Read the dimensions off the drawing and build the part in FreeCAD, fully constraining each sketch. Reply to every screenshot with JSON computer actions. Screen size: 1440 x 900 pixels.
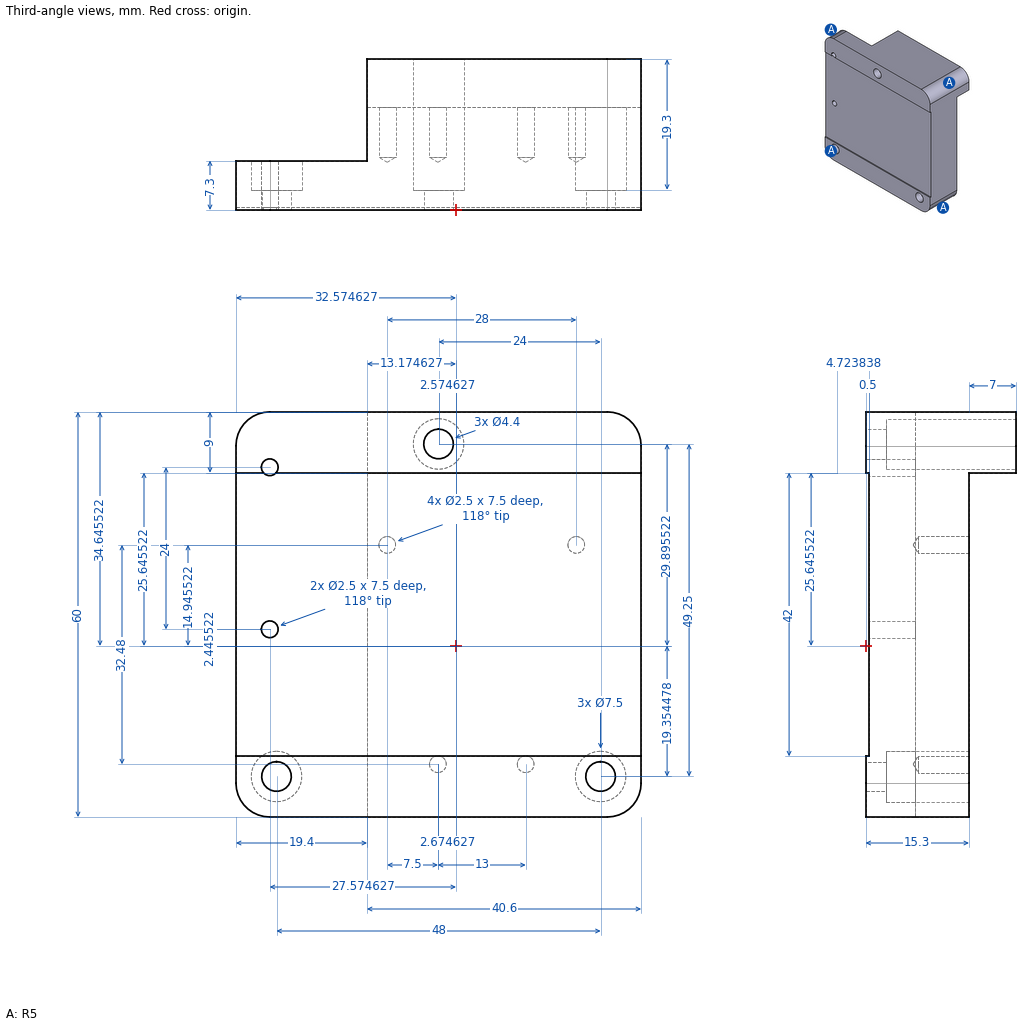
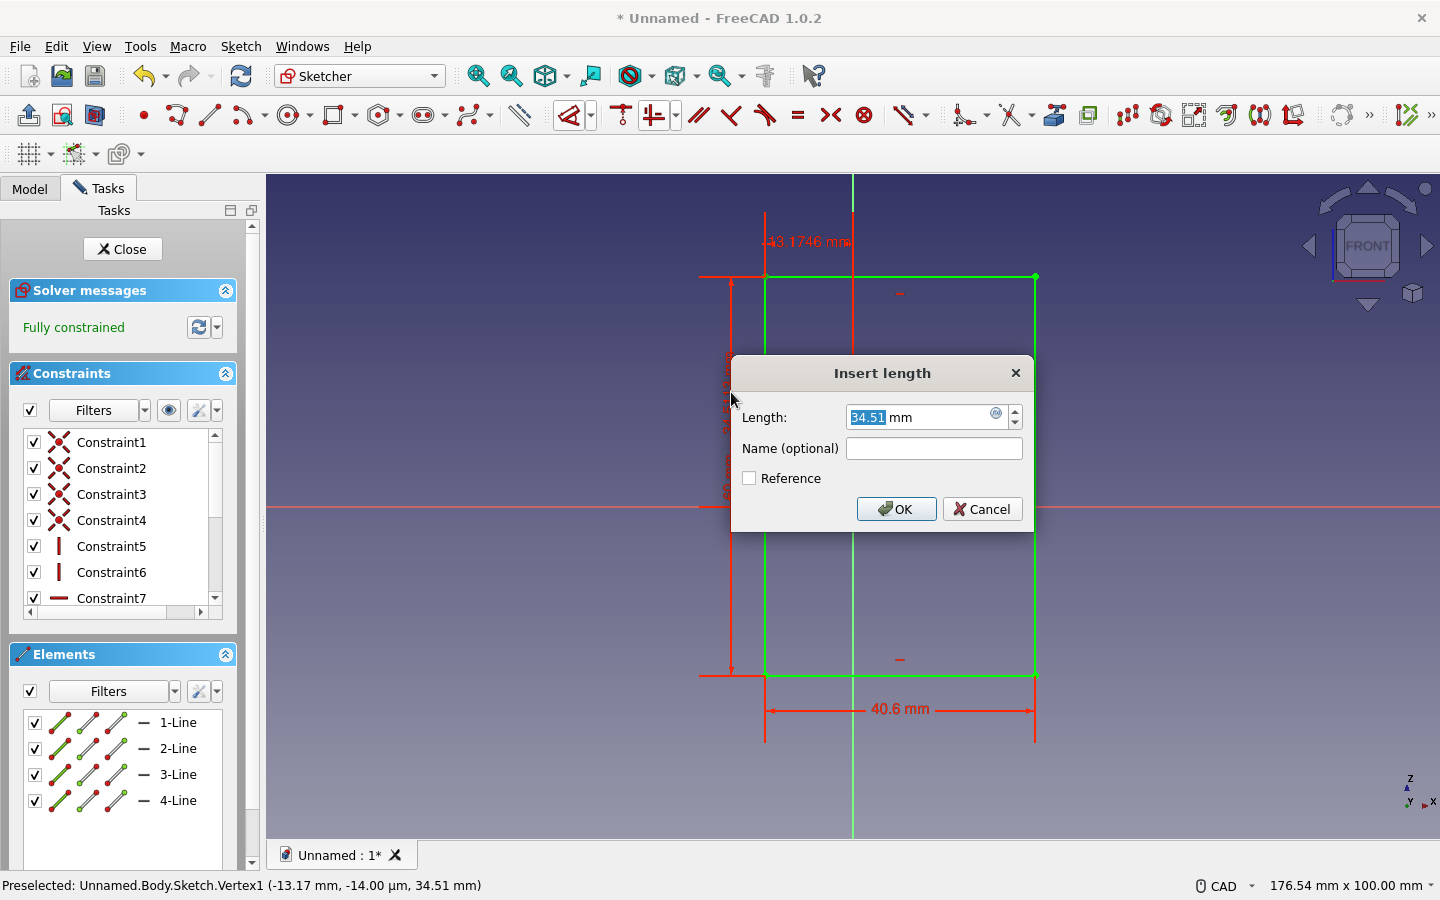
{"action": "type", "text": "34.645522"}
{"action": "key", "text": "Return"}
{"action": "key", "text": "Escape"}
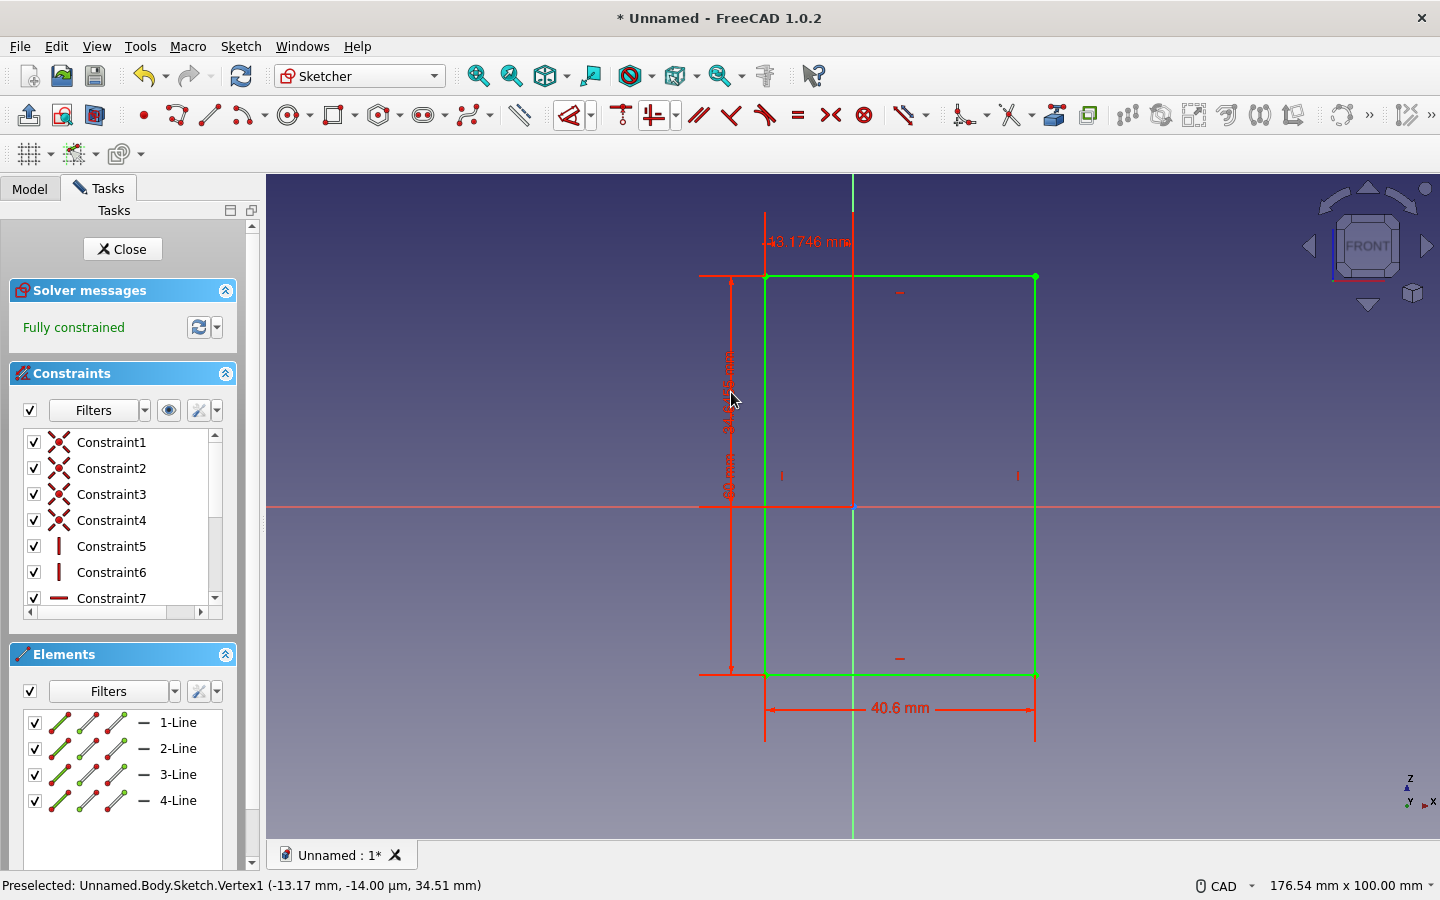
{"action": "left_click", "coordinate": [123, 249]}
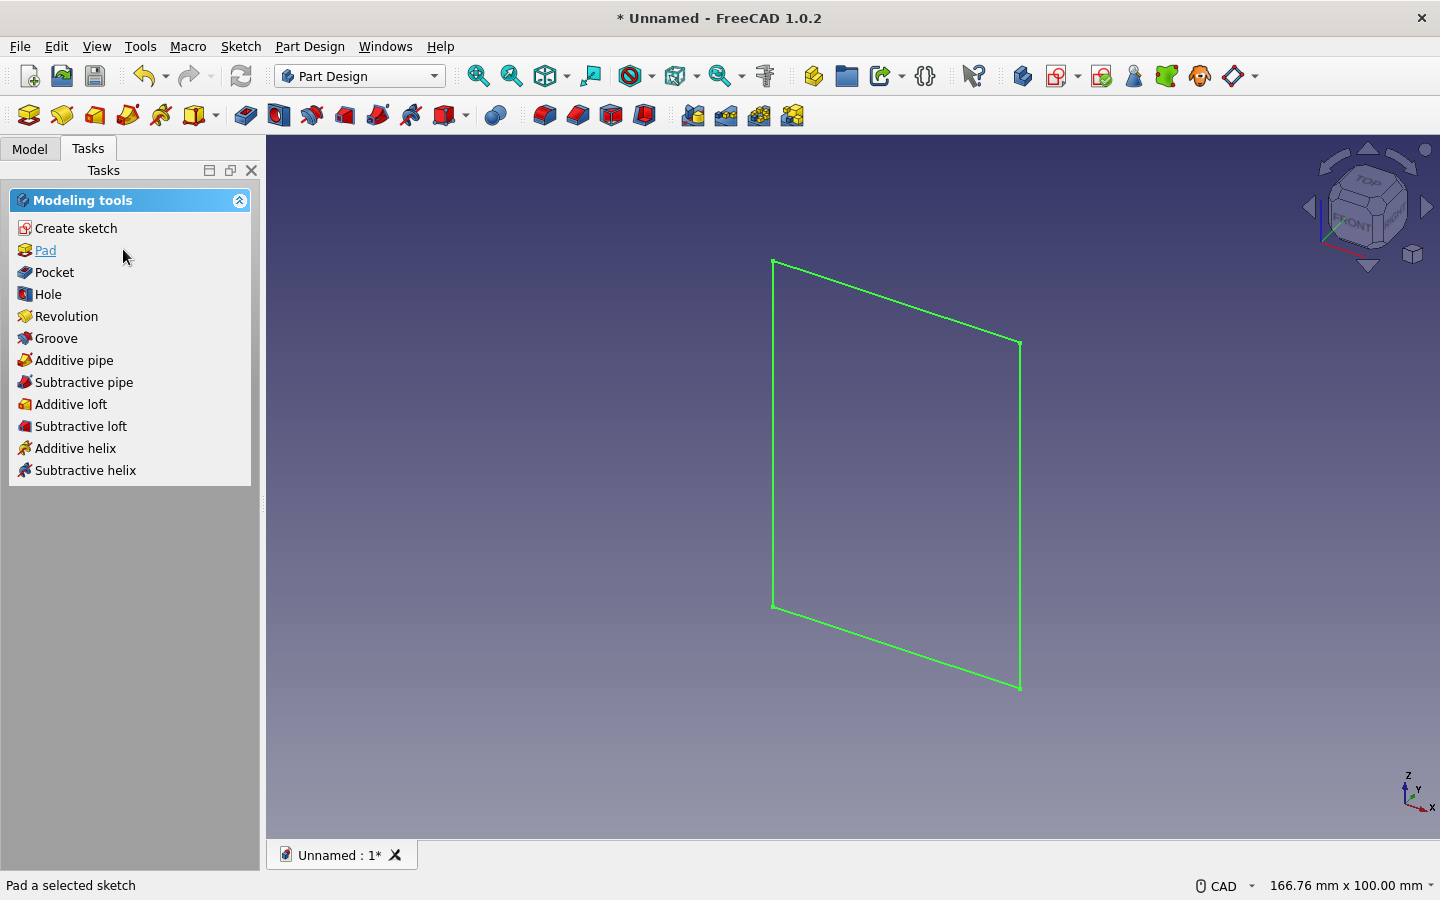
{"action": "left_click", "coordinate": [29, 116]}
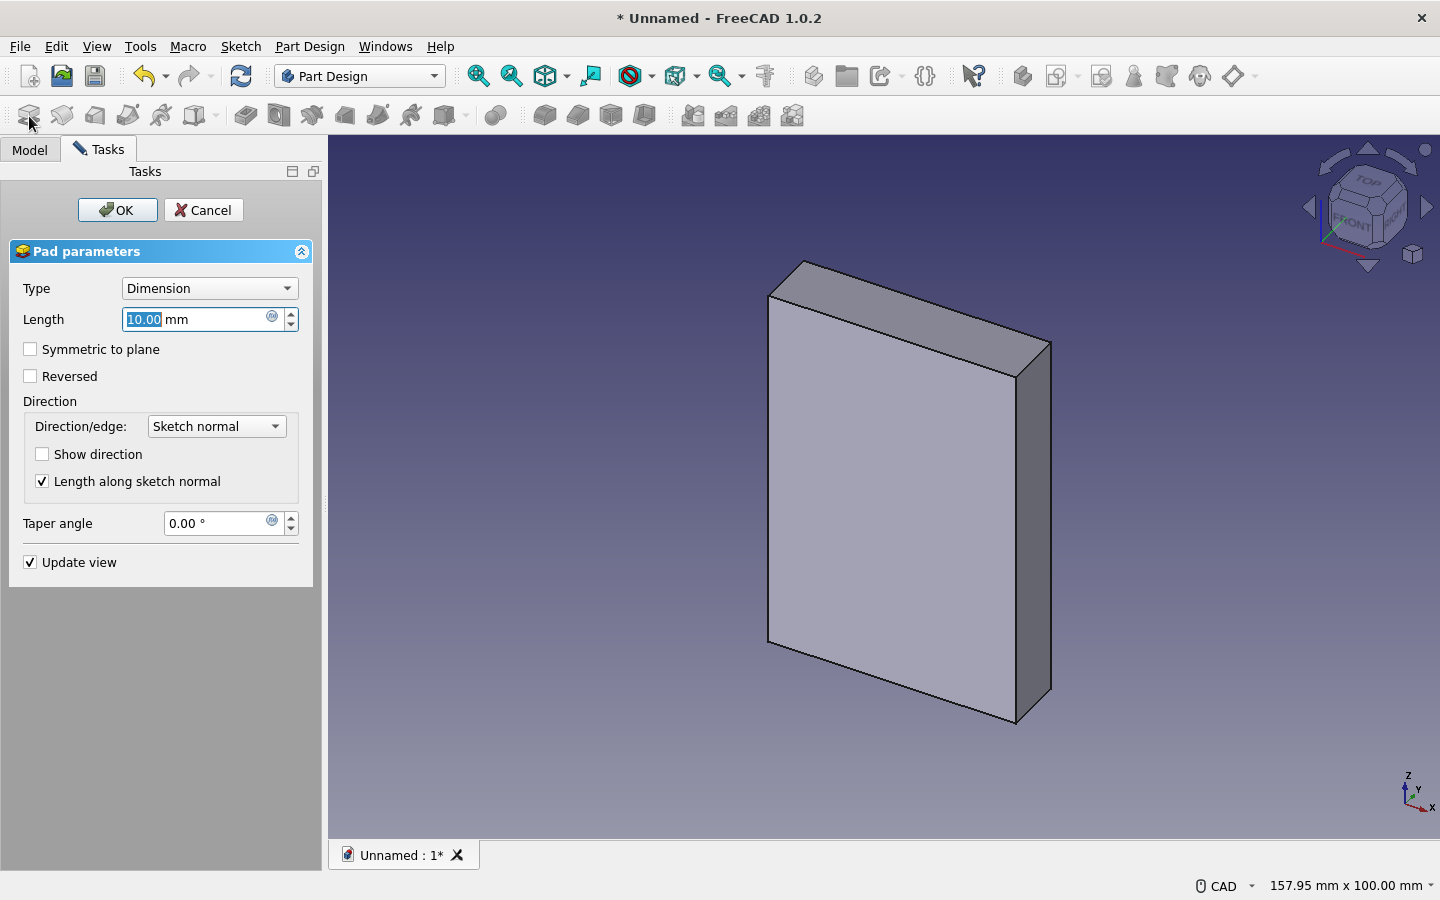
{"action": "type", "text": "15.3"}
{"action": "key", "text": "Tab"}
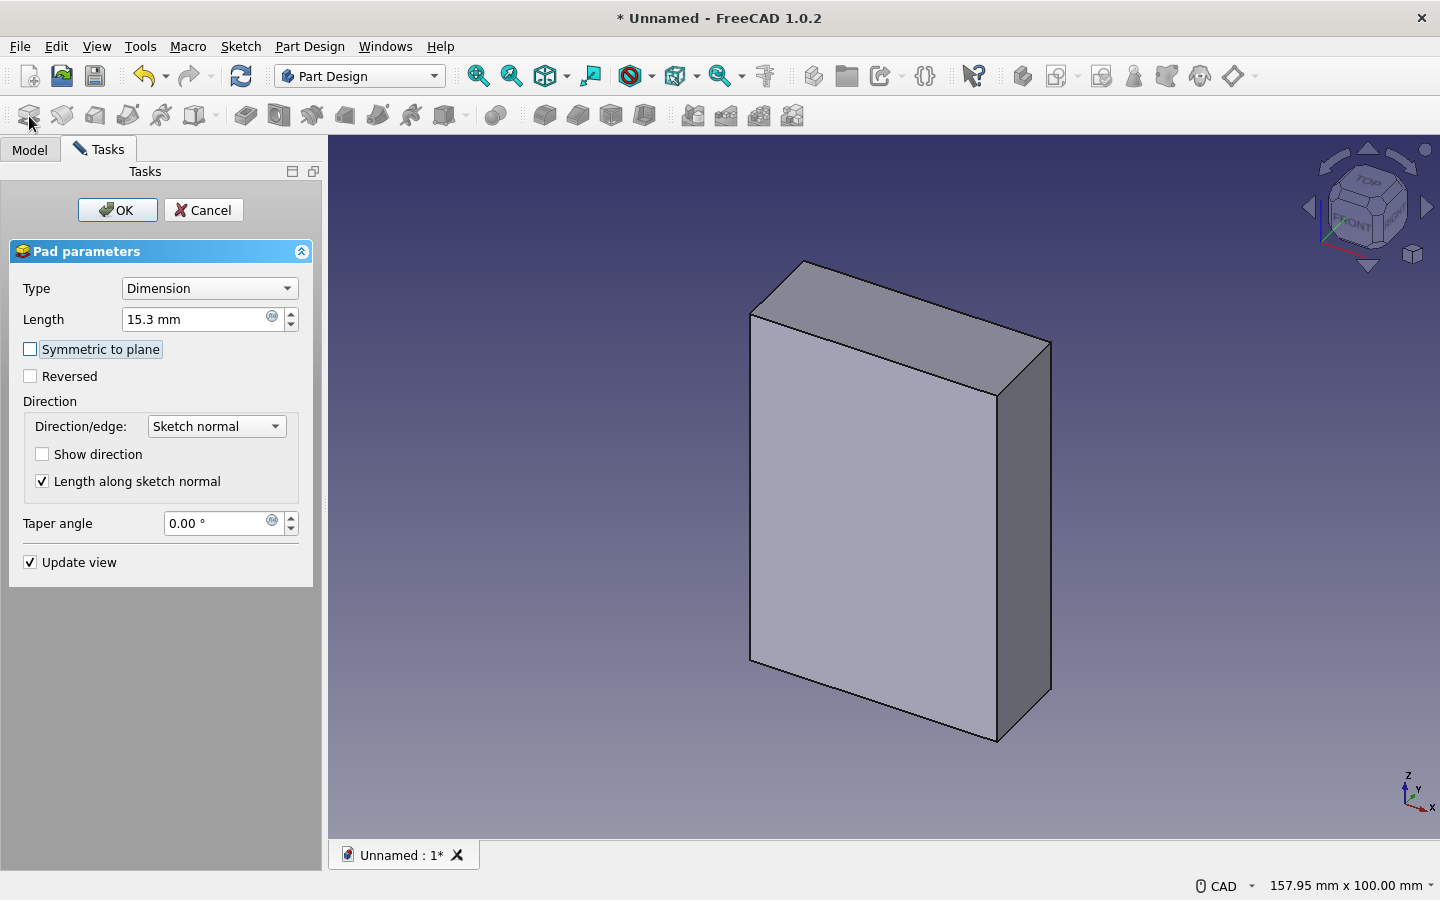
{"action": "left_click", "coordinate": [31, 376]}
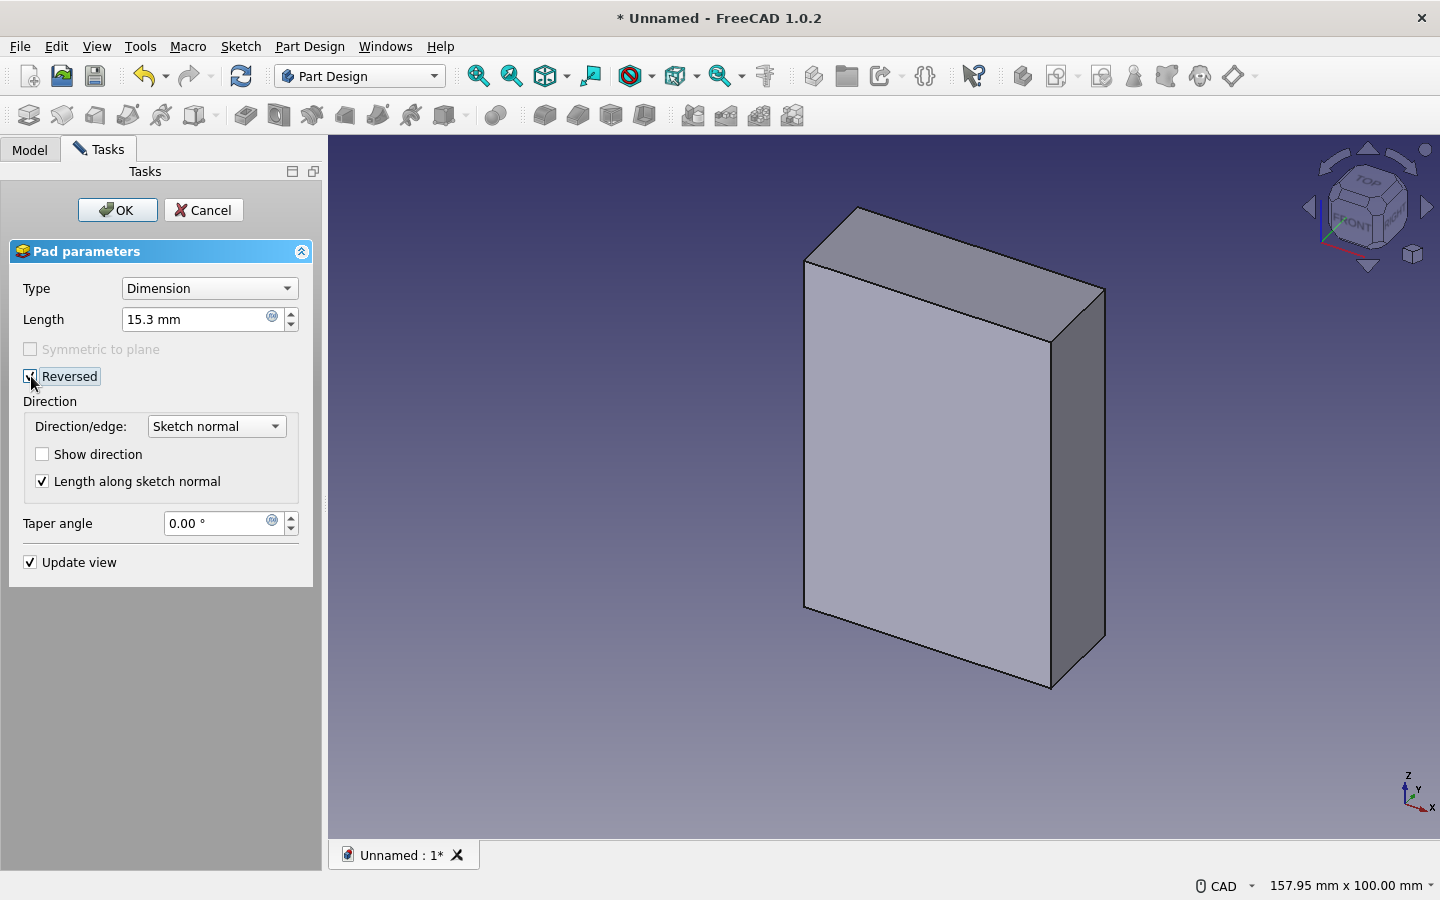
{"action": "left_click", "coordinate": [118, 210]}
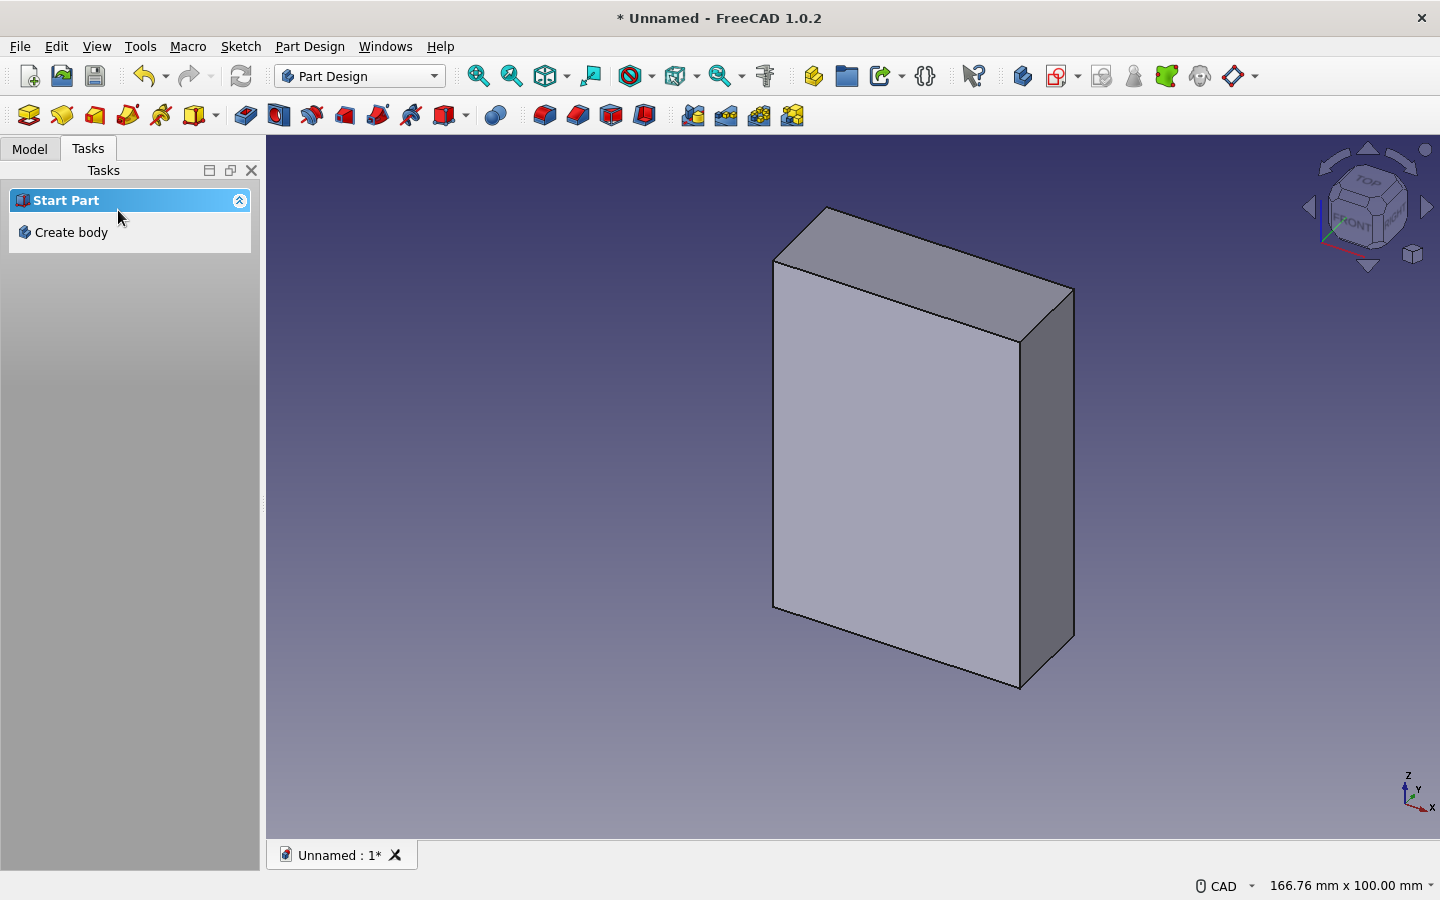
{"action": "left_click", "coordinate": [1056, 76]}